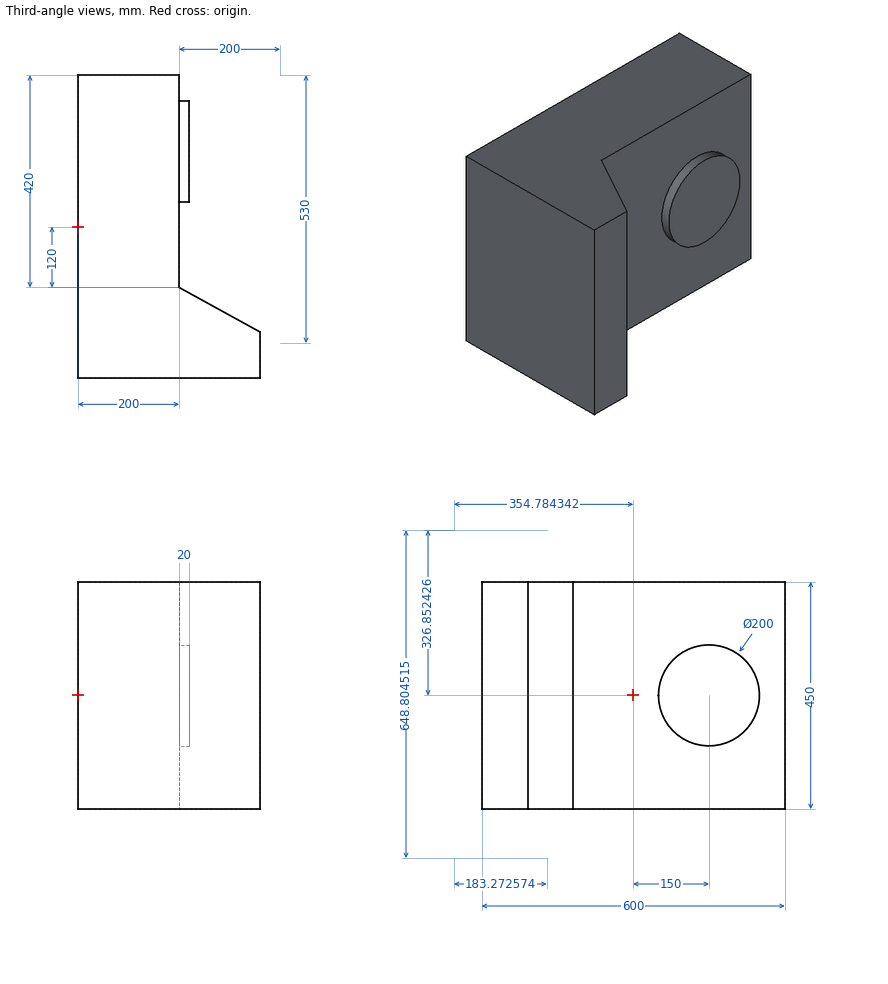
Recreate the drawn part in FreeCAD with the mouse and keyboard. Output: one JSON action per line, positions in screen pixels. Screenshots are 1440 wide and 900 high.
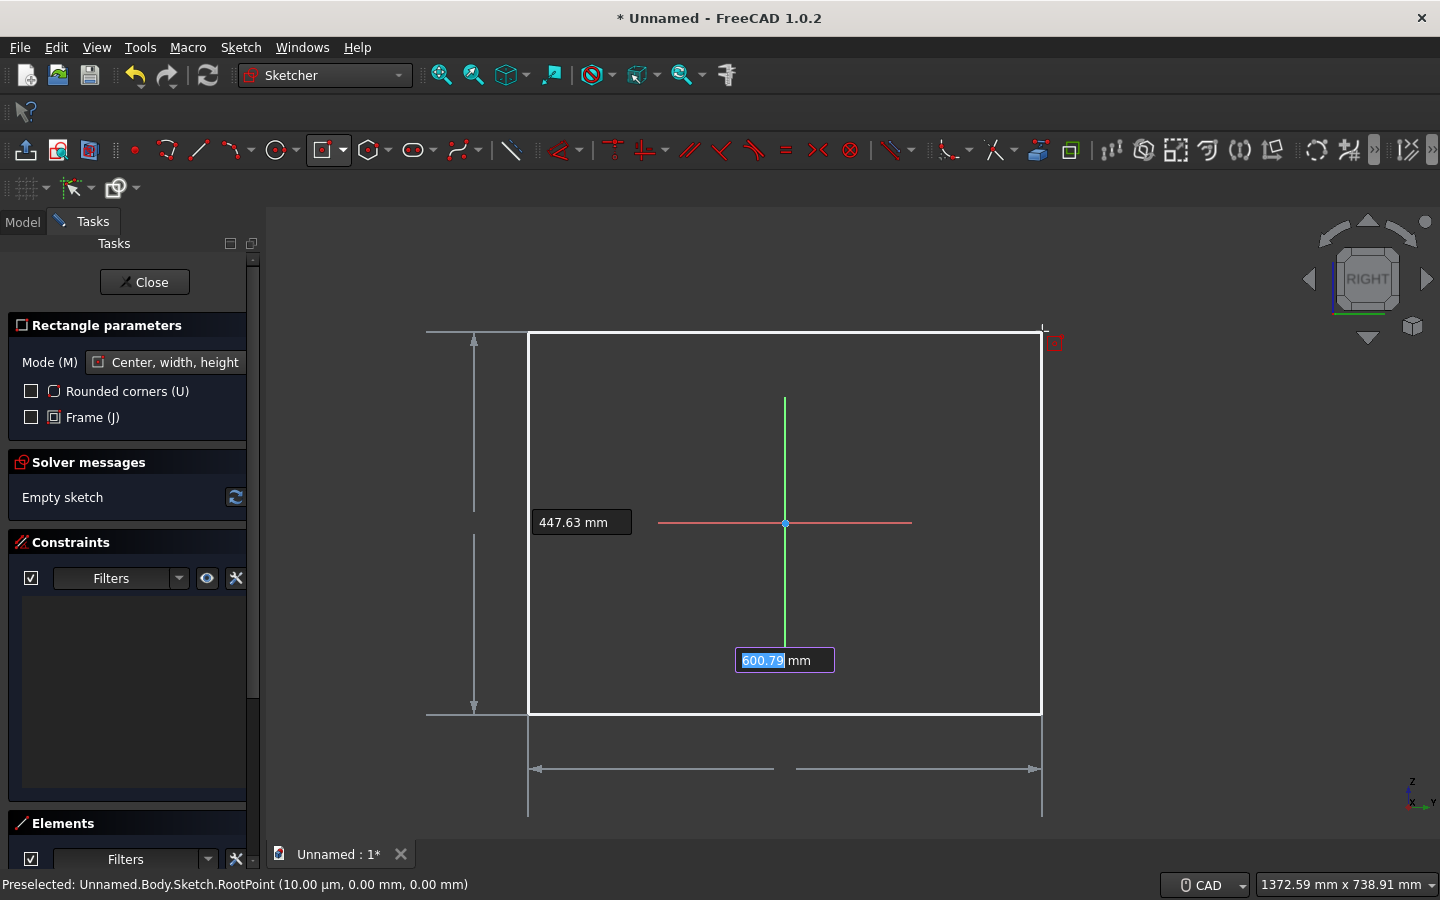
{"action": "type", "text": "600"}
{"action": "key", "text": "Tab"}
{"action": "type", "text": "450"}
{"action": "key", "text": "Return"}
{"action": "key", "text": "Escape"}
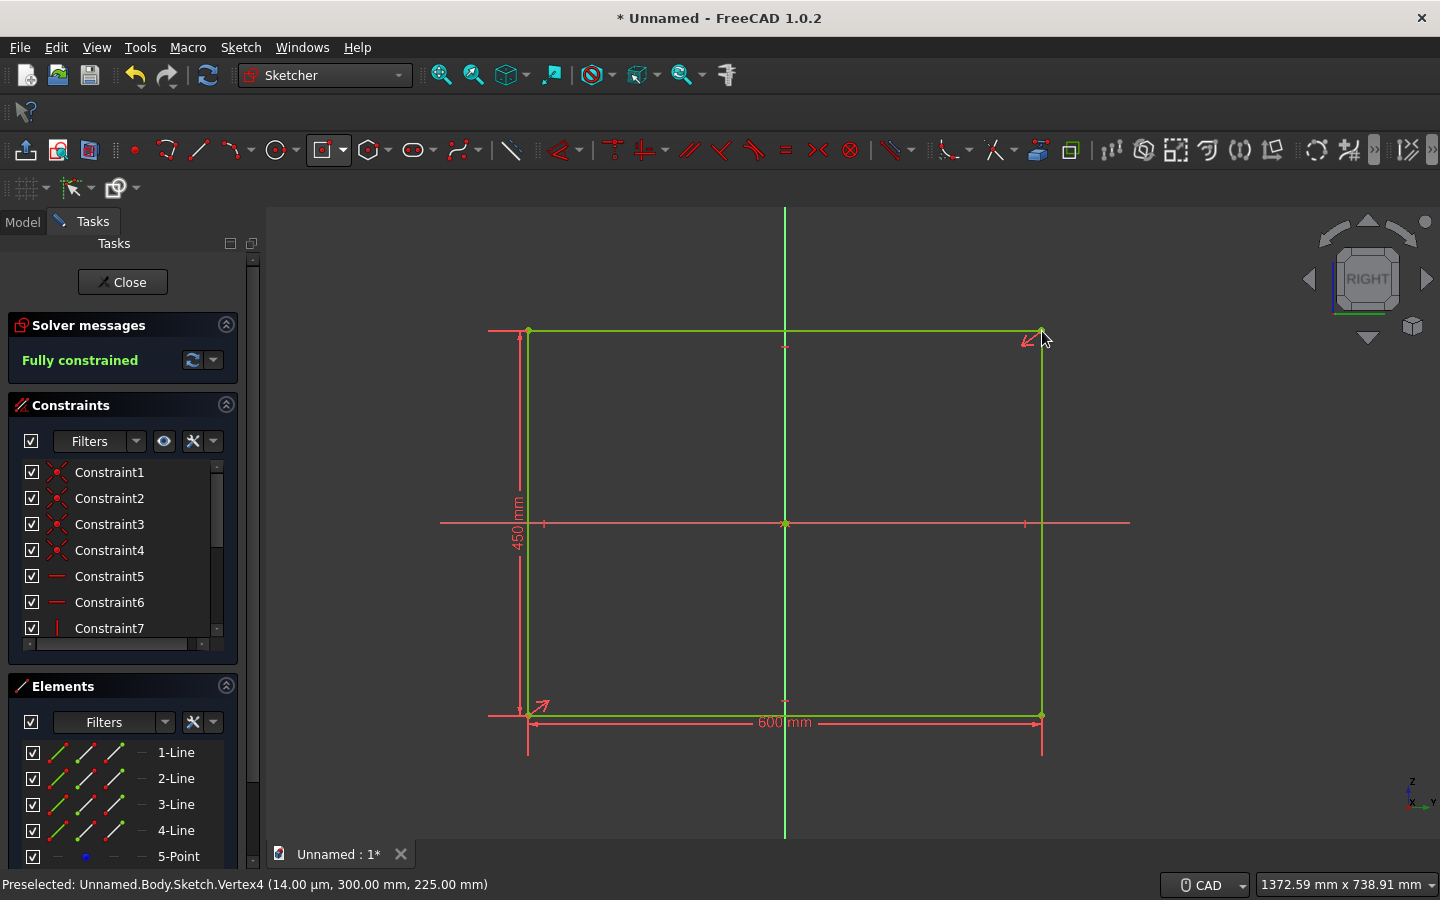
{"action": "left_click", "coordinate": [123, 282]}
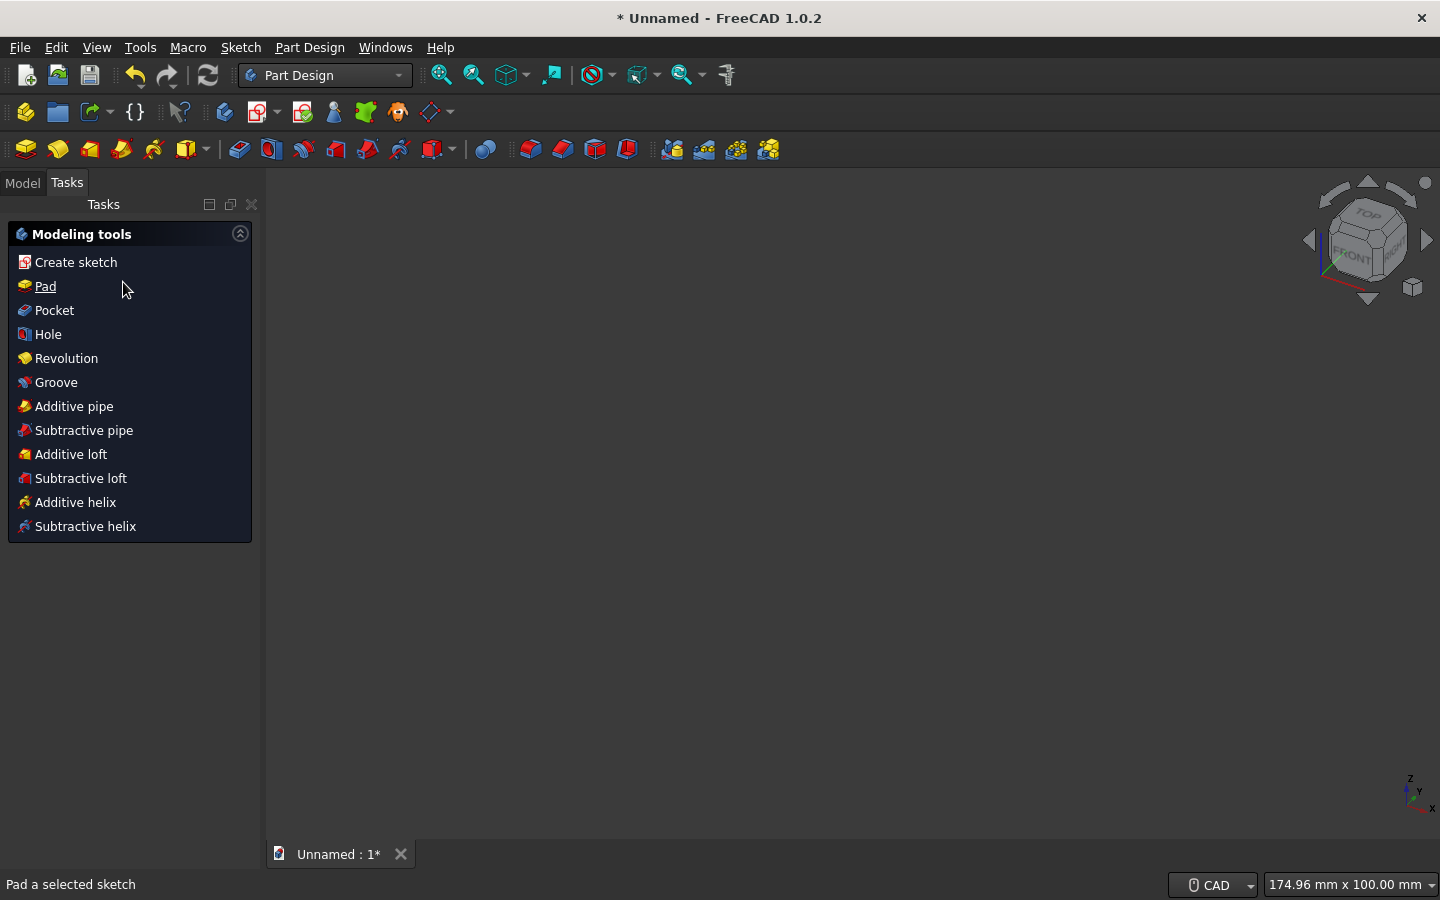
{"action": "left_click", "coordinate": [26, 150]}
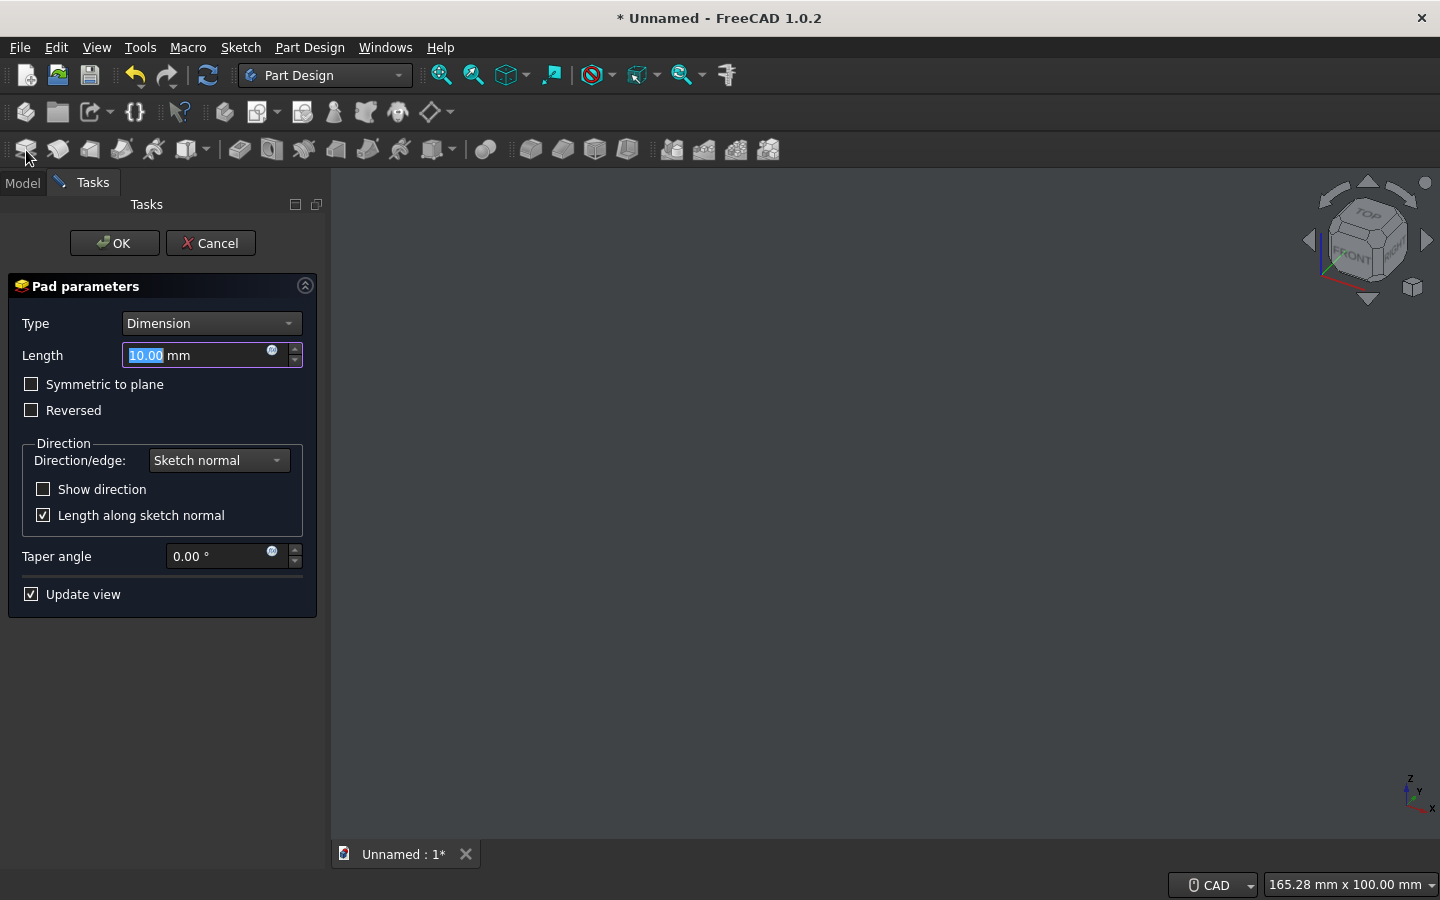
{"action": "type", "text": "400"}
{"action": "key", "text": "Tab"}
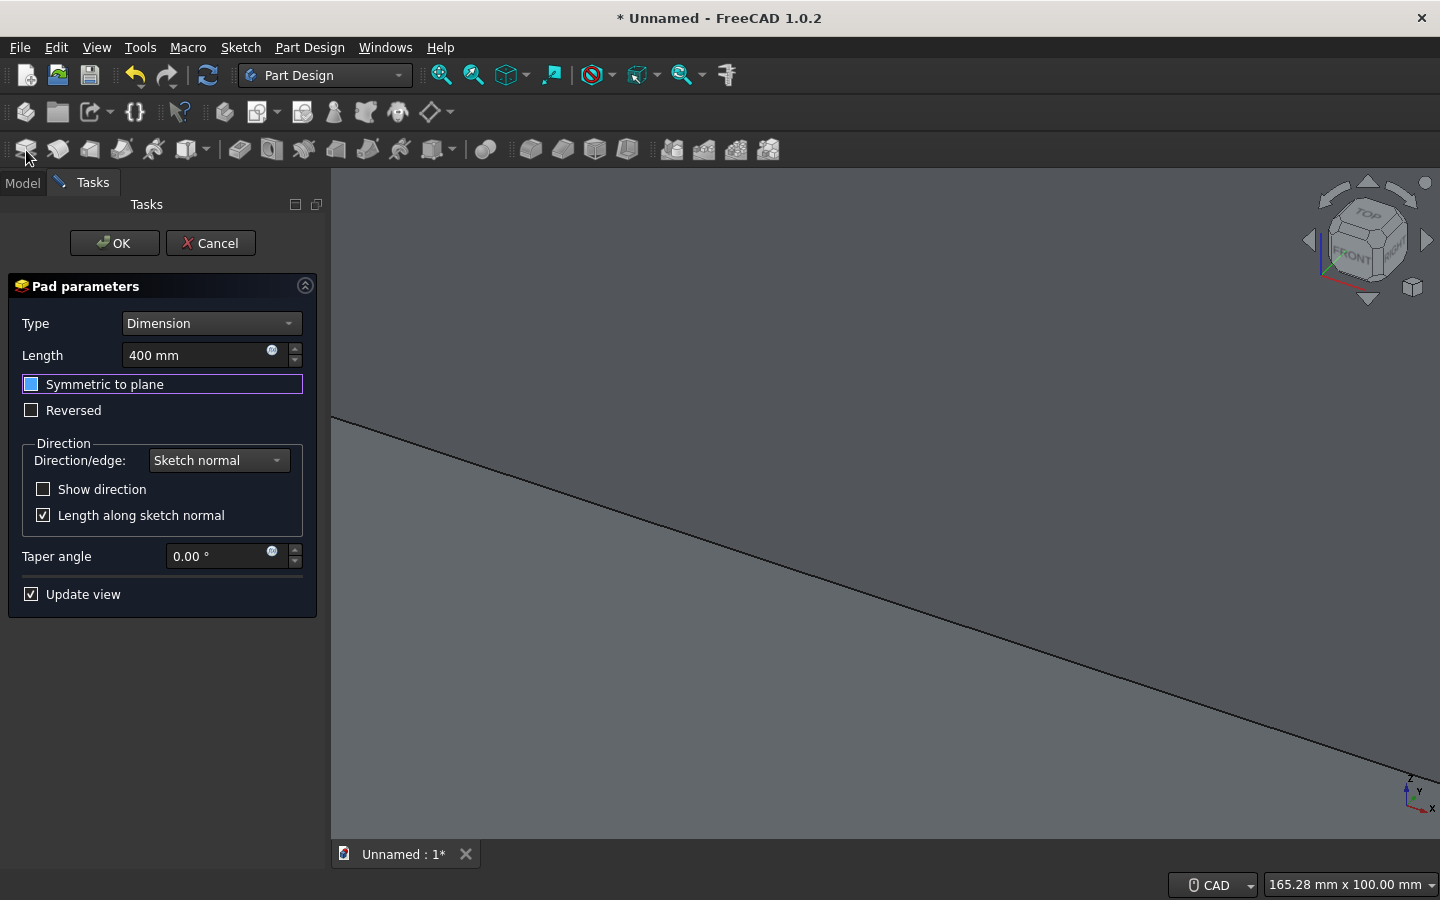
{"action": "left_click", "coordinate": [115, 243]}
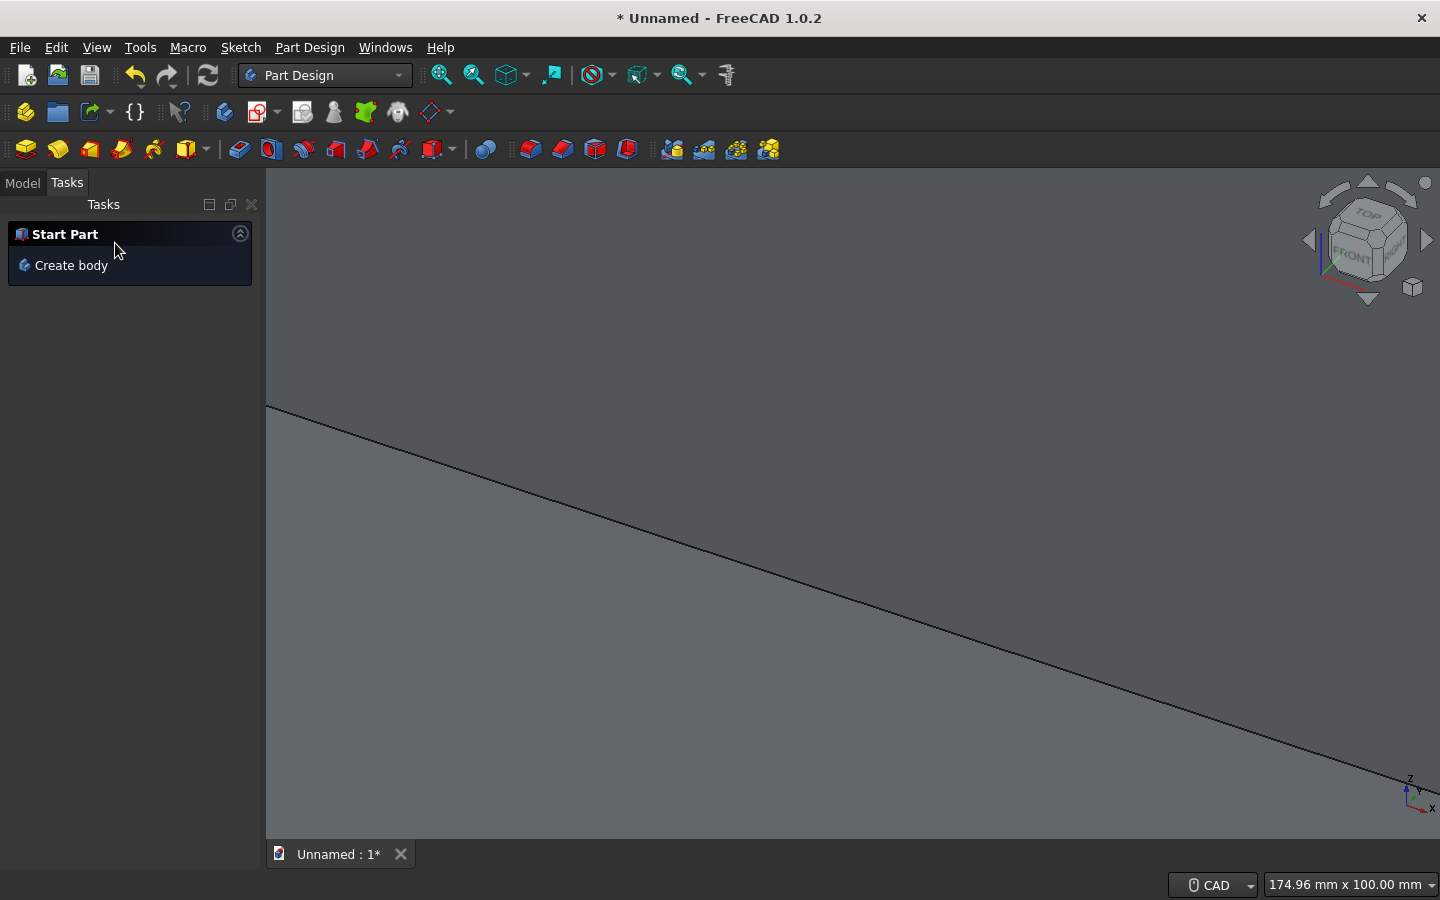
{"action": "left_click", "coordinate": [442, 76]}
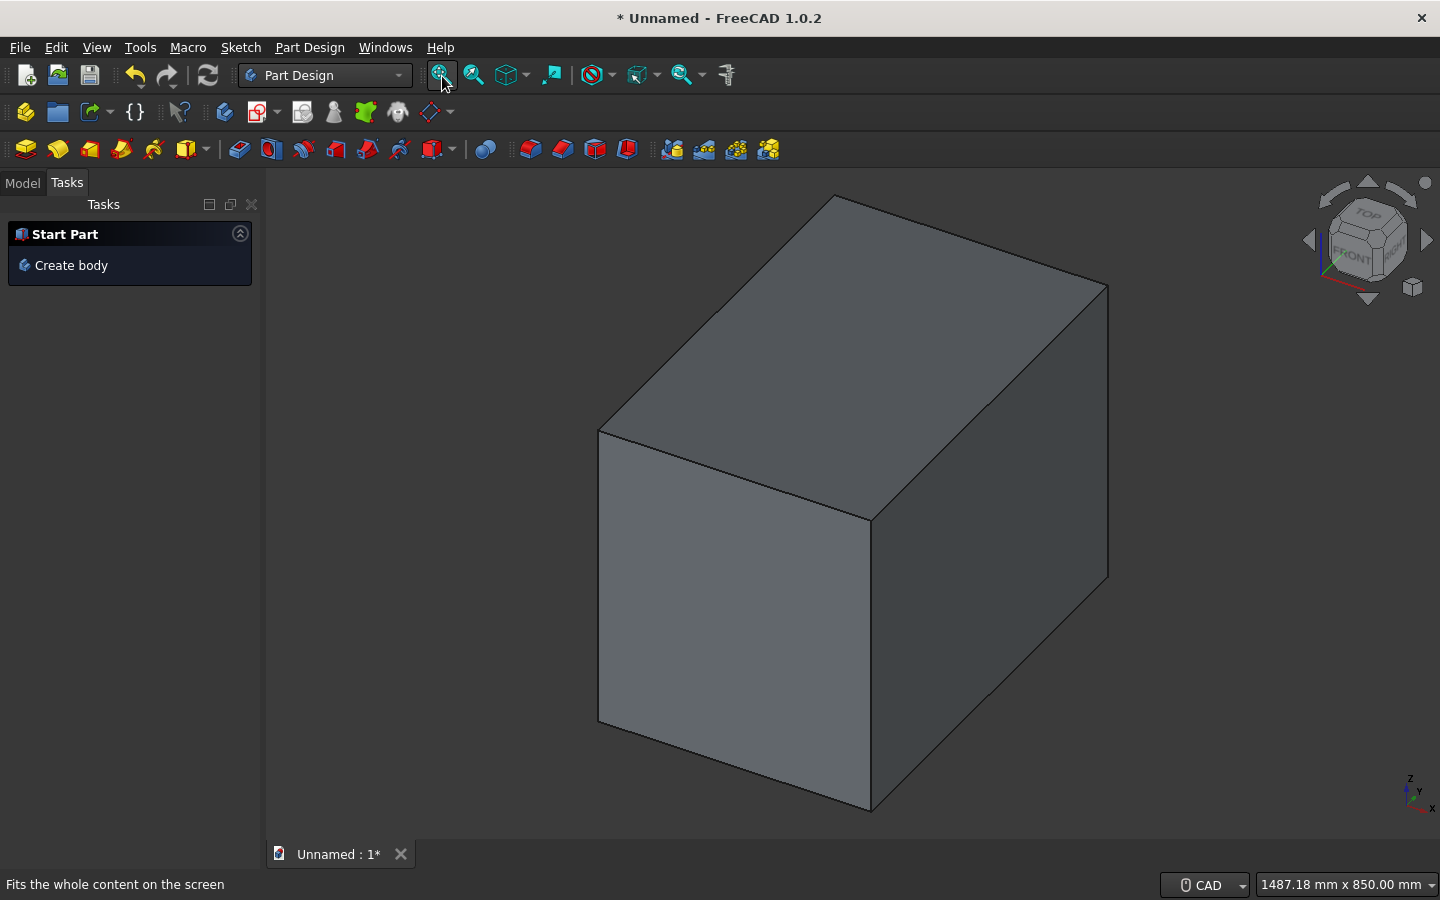
{"action": "left_click", "coordinate": [887, 323]}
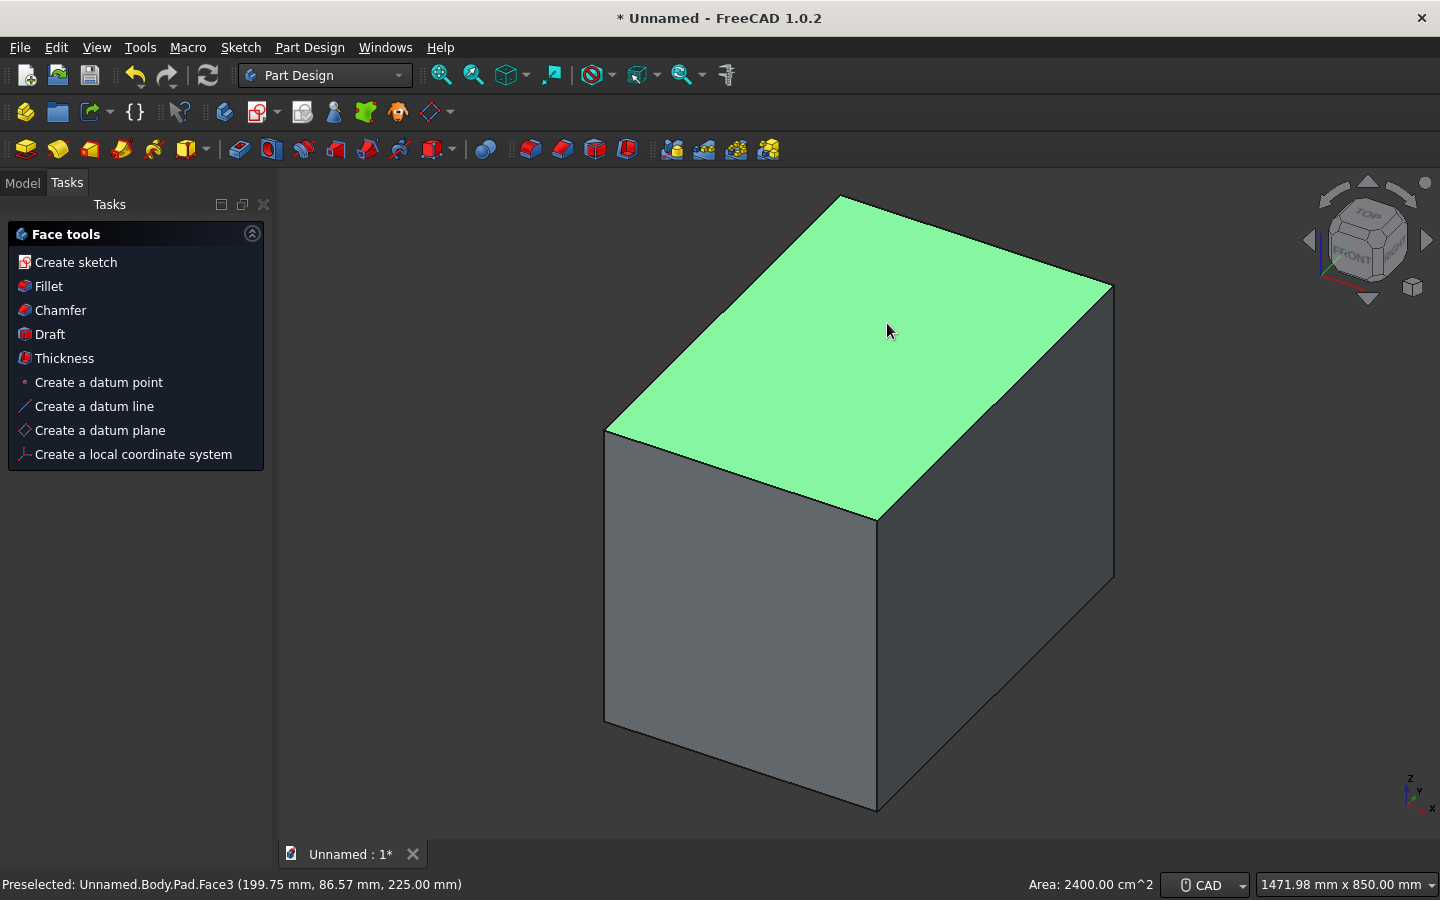
{"action": "left_click", "coordinate": [258, 112]}